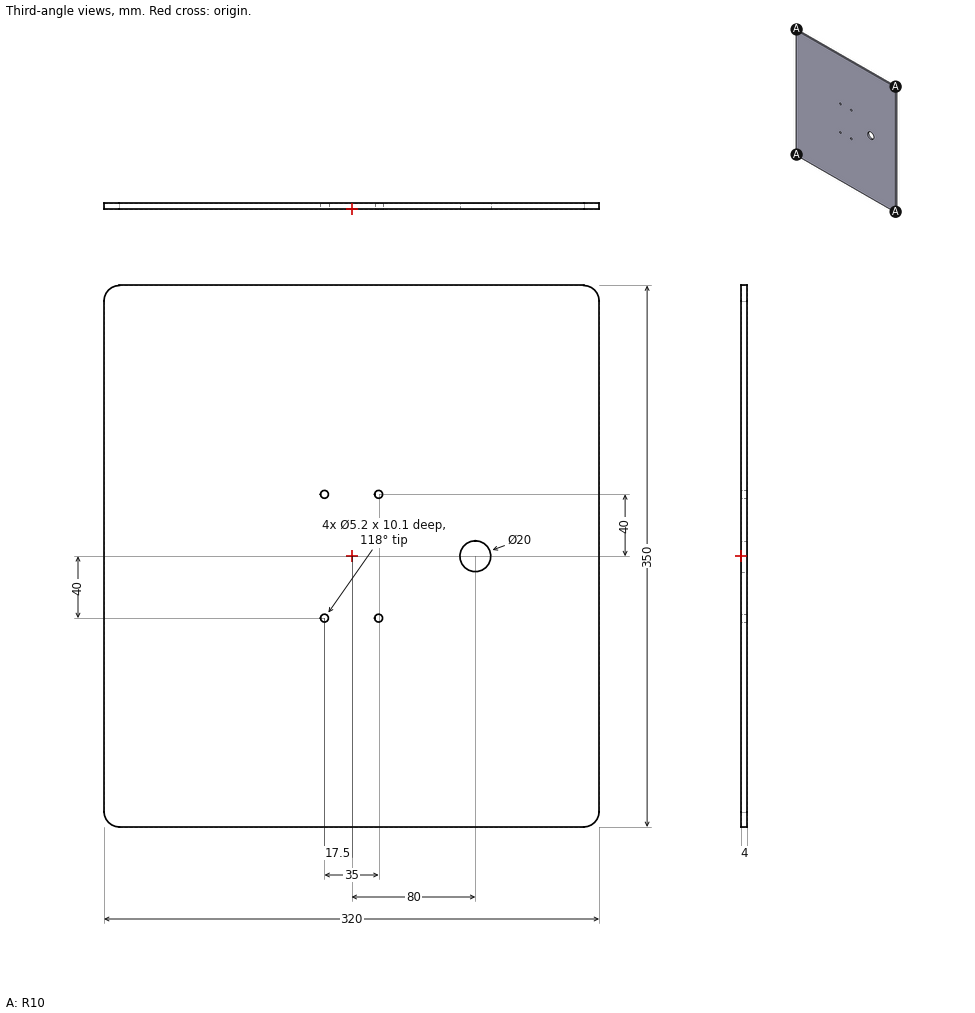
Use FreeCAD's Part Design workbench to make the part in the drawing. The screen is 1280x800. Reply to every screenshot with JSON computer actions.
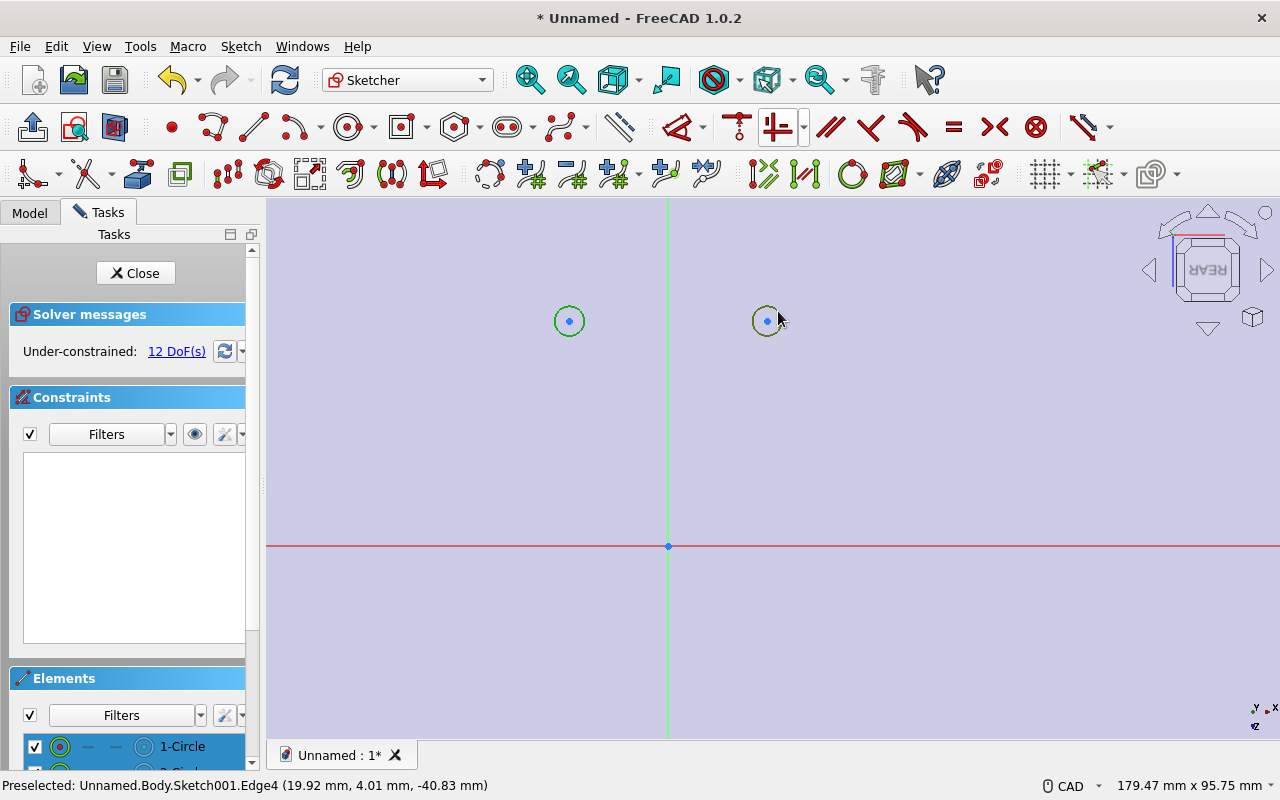
{"action": "left_click", "coordinate": [954, 128]}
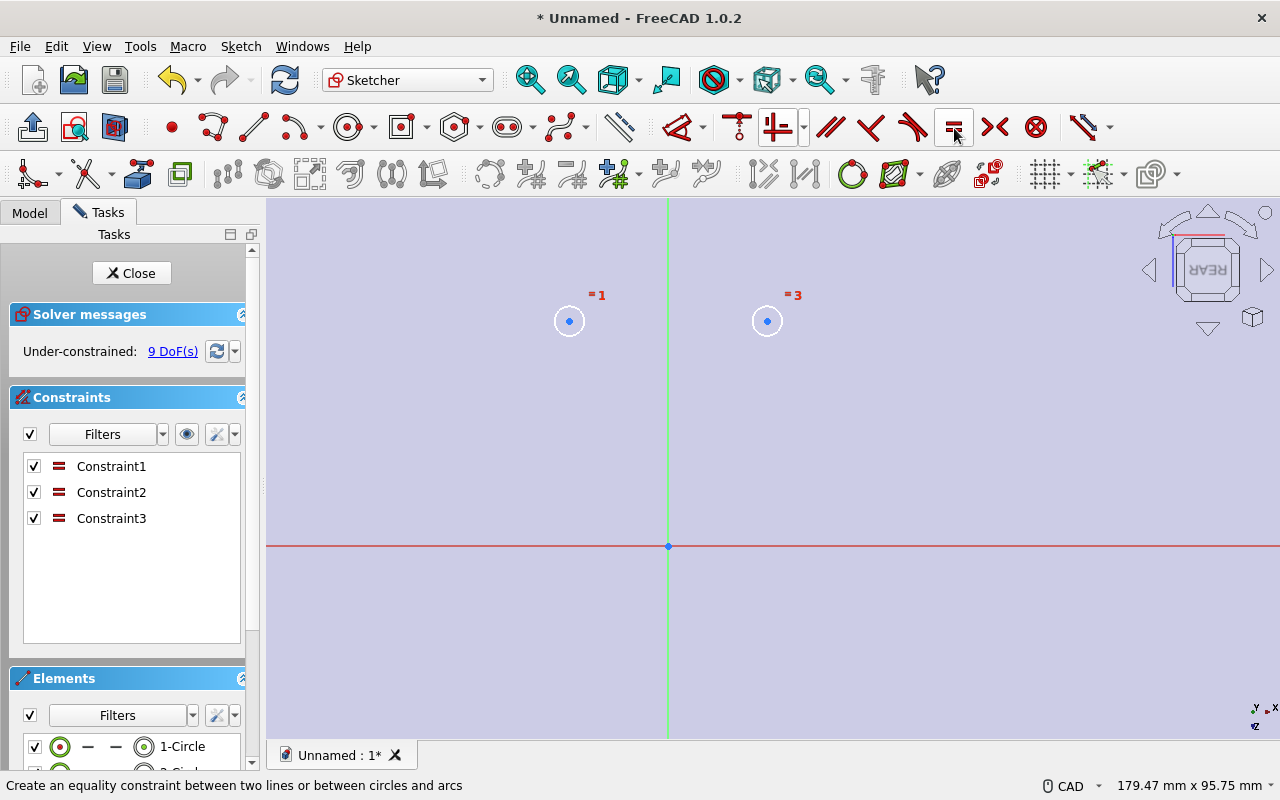
{"action": "left_click", "coordinate": [569, 321]}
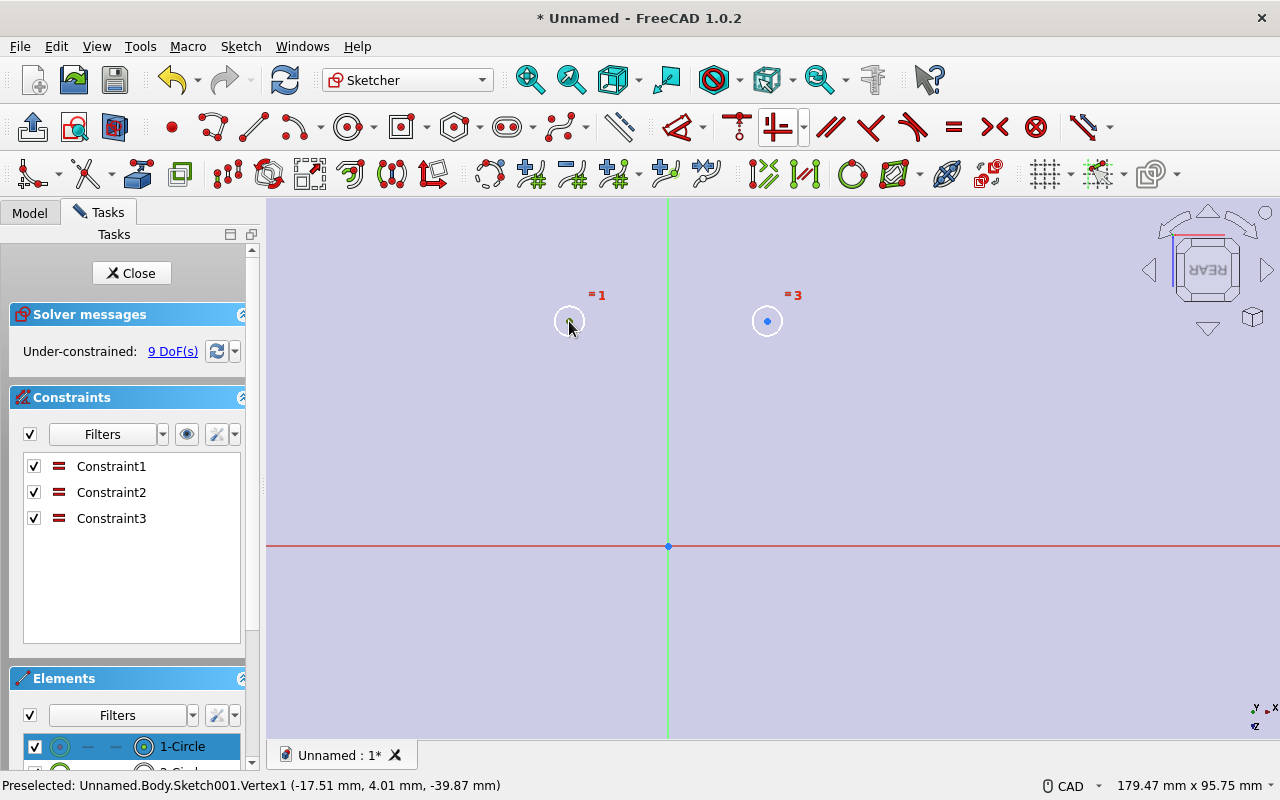
{"action": "scroll", "coordinate": [778, 310], "scroll_direction": "down", "scroll_amount": 2}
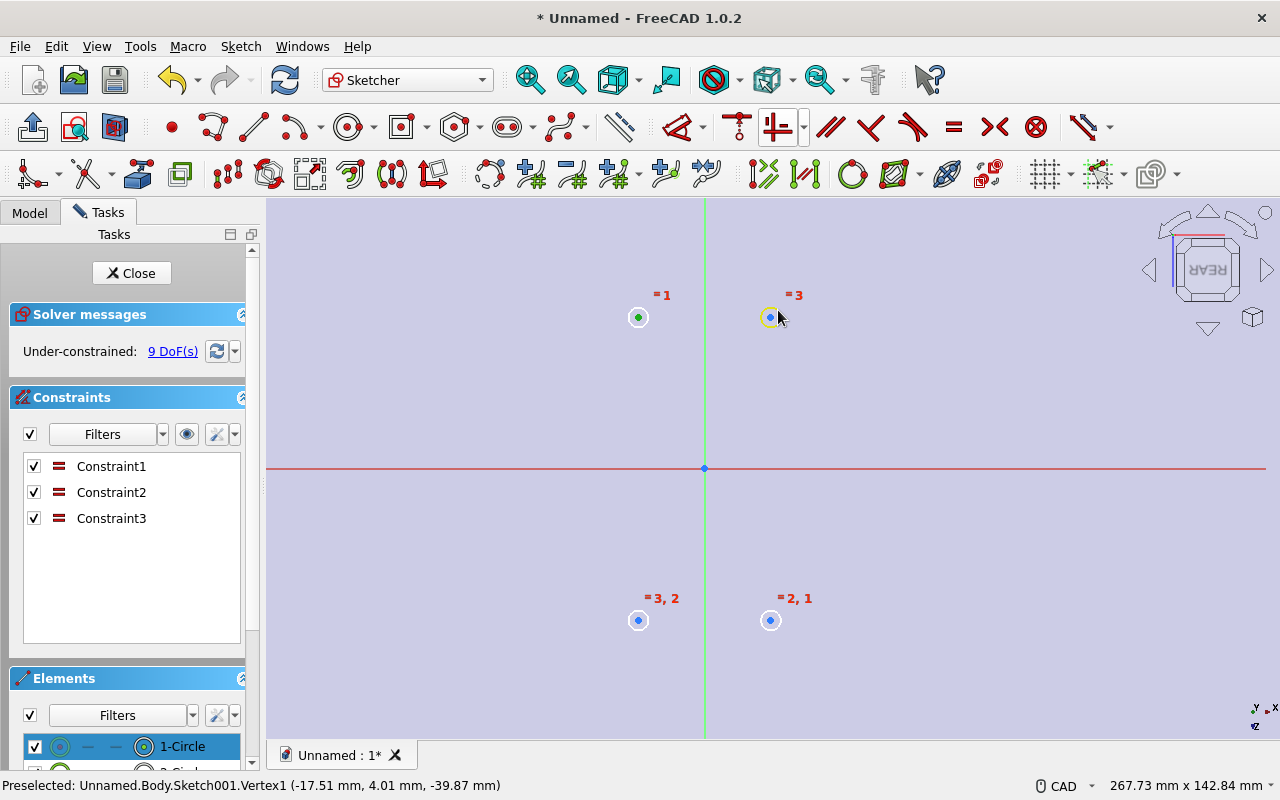
{"action": "left_click", "coordinate": [639, 620]}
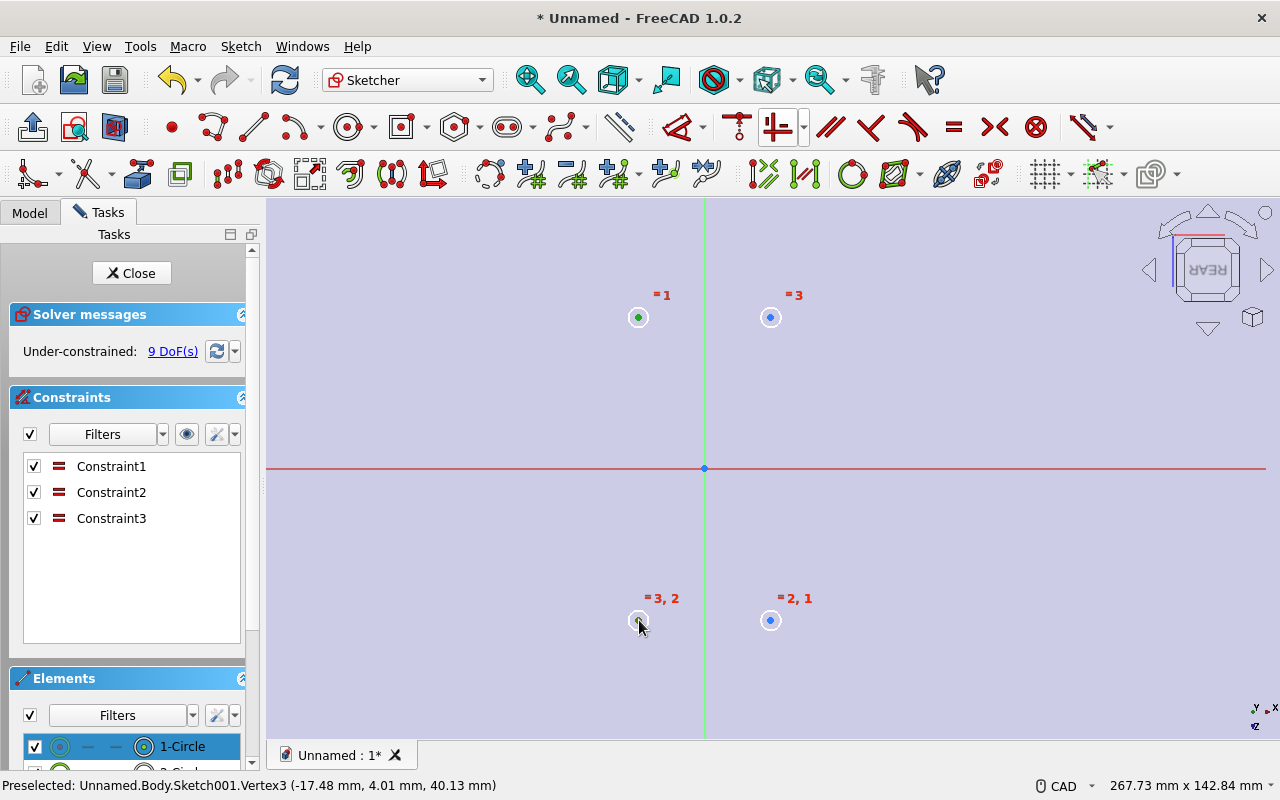
{"action": "key", "text": "v"}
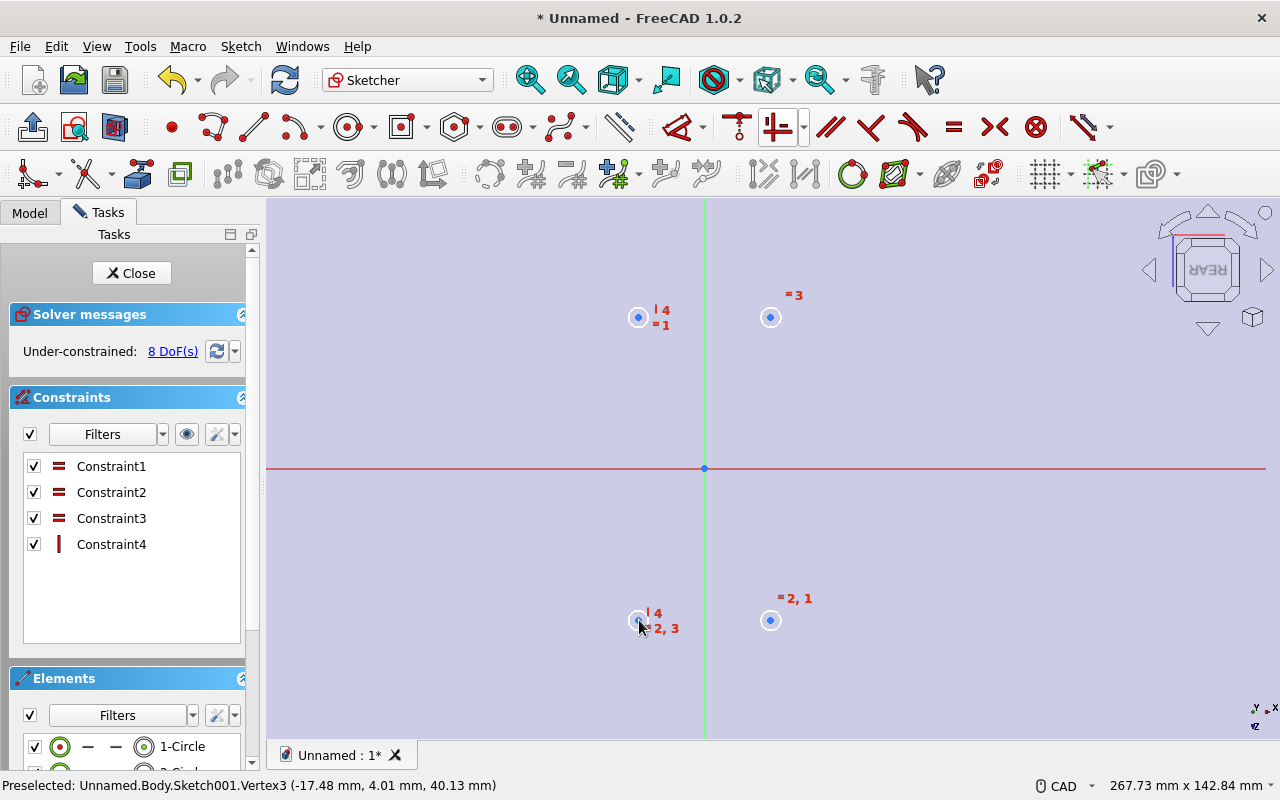
{"action": "left_click", "coordinate": [771, 620]}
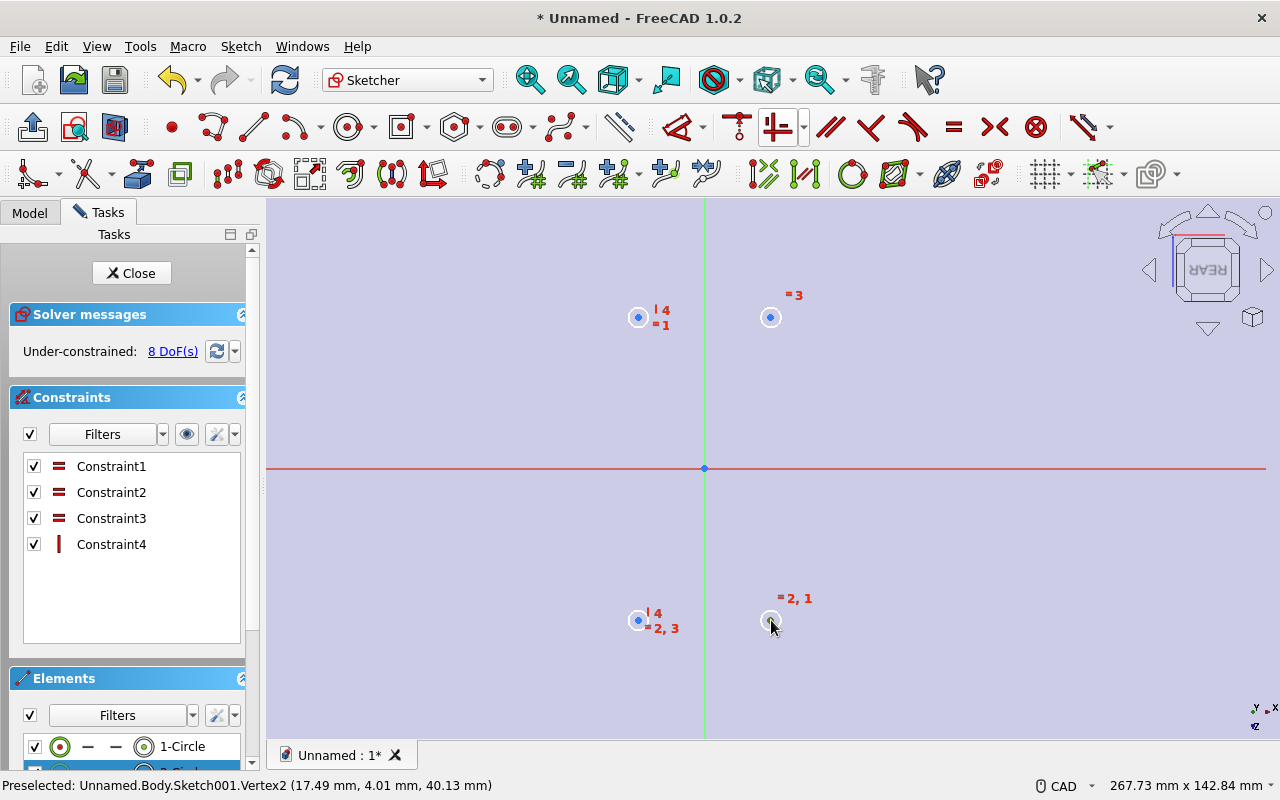
{"action": "left_click", "coordinate": [638, 620]}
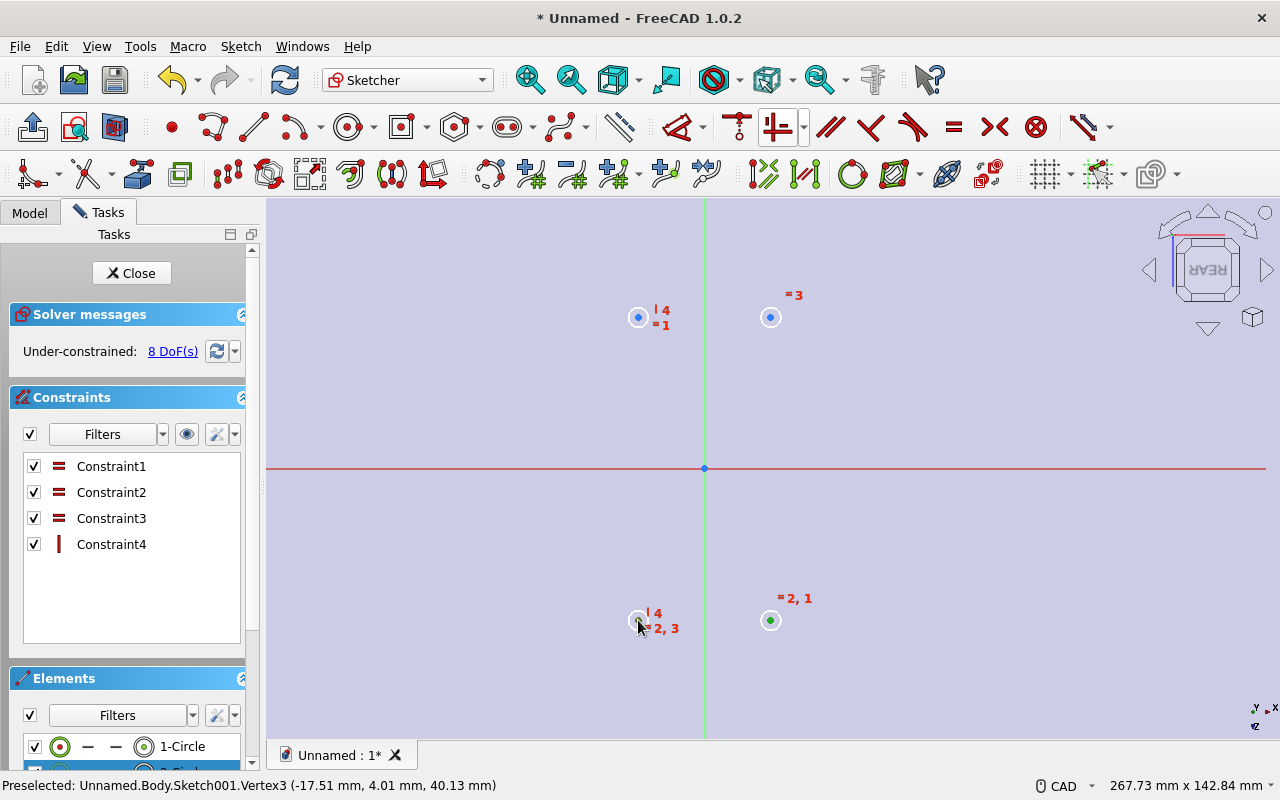
{"action": "key", "text": "h"}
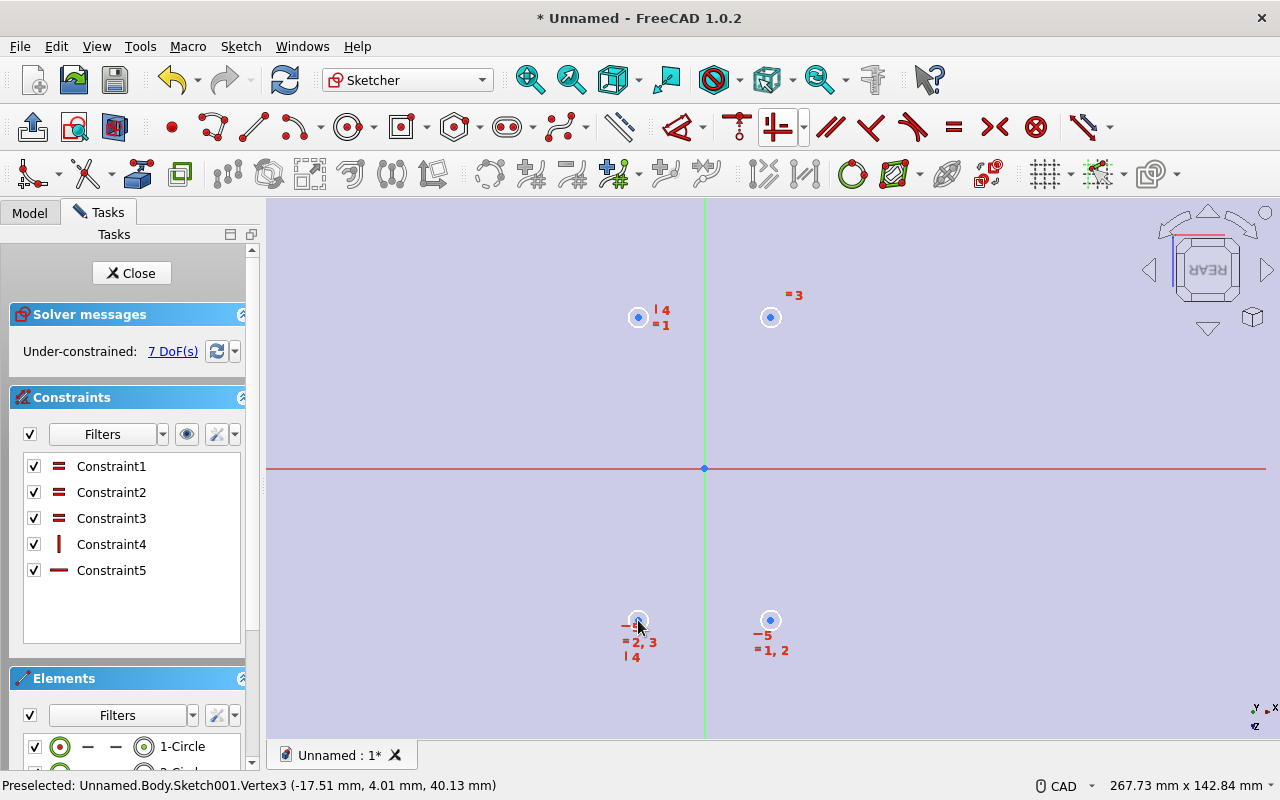
{"action": "left_click", "coordinate": [771, 620]}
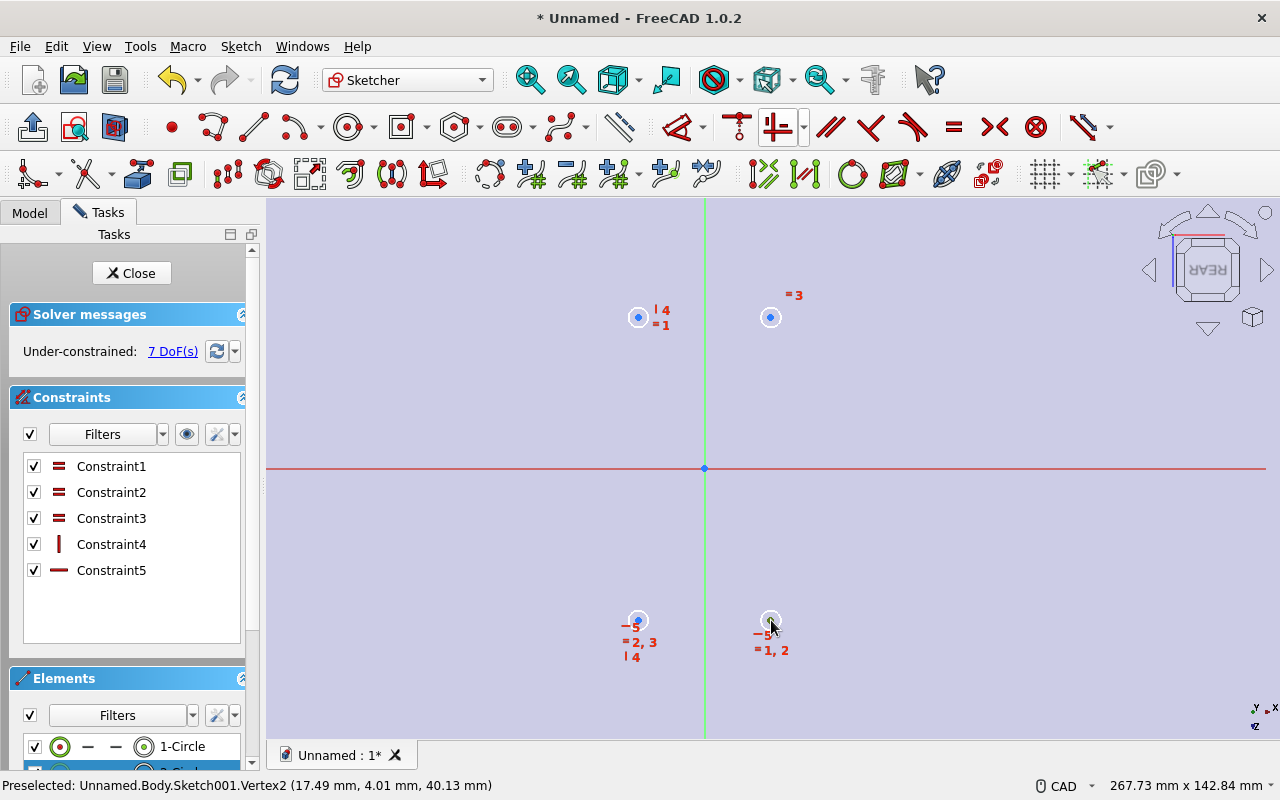
{"action": "left_click", "coordinate": [771, 318]}